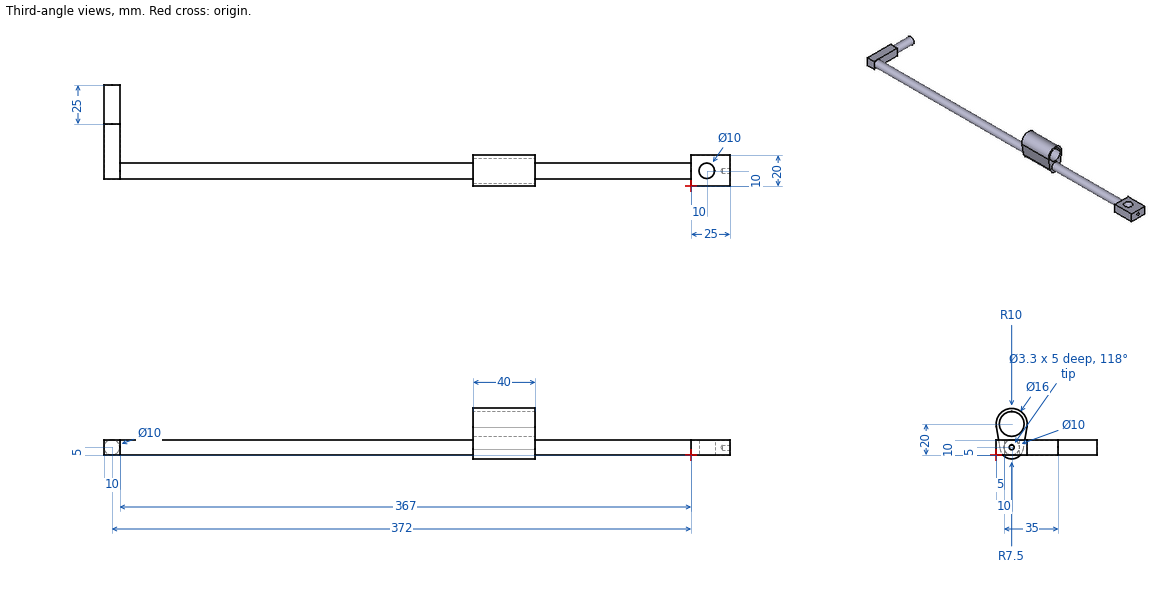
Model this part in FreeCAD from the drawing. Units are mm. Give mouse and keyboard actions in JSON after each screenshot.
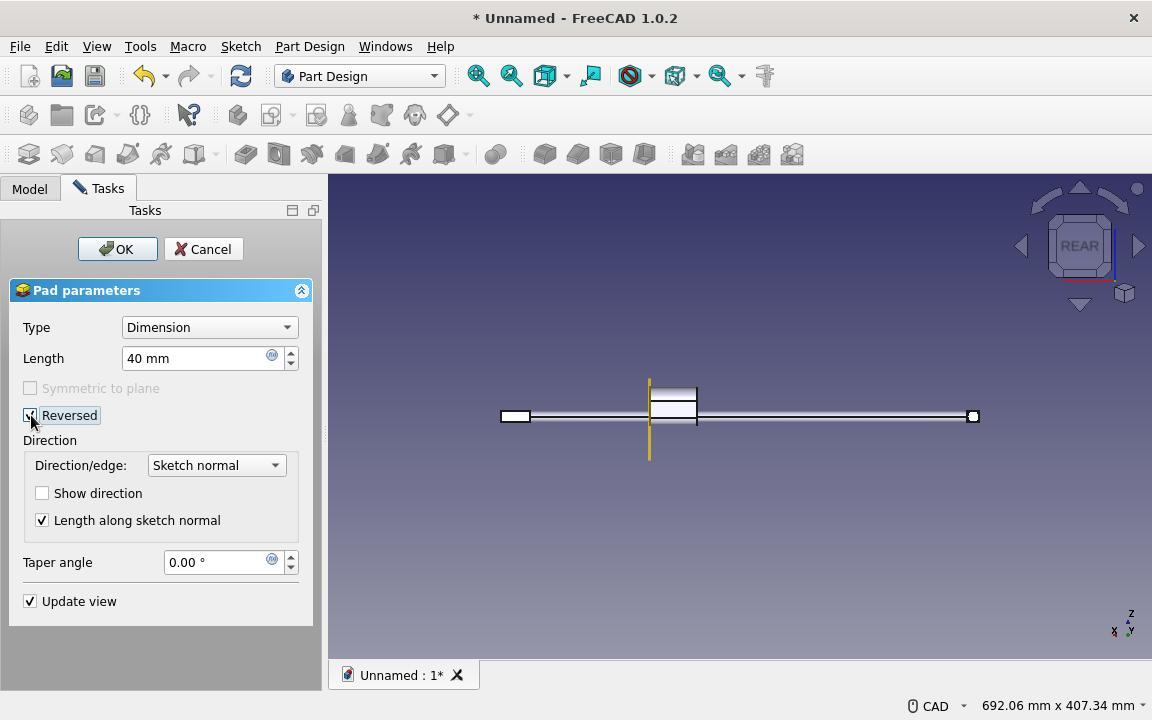
{"action": "left_click", "coordinate": [118, 249]}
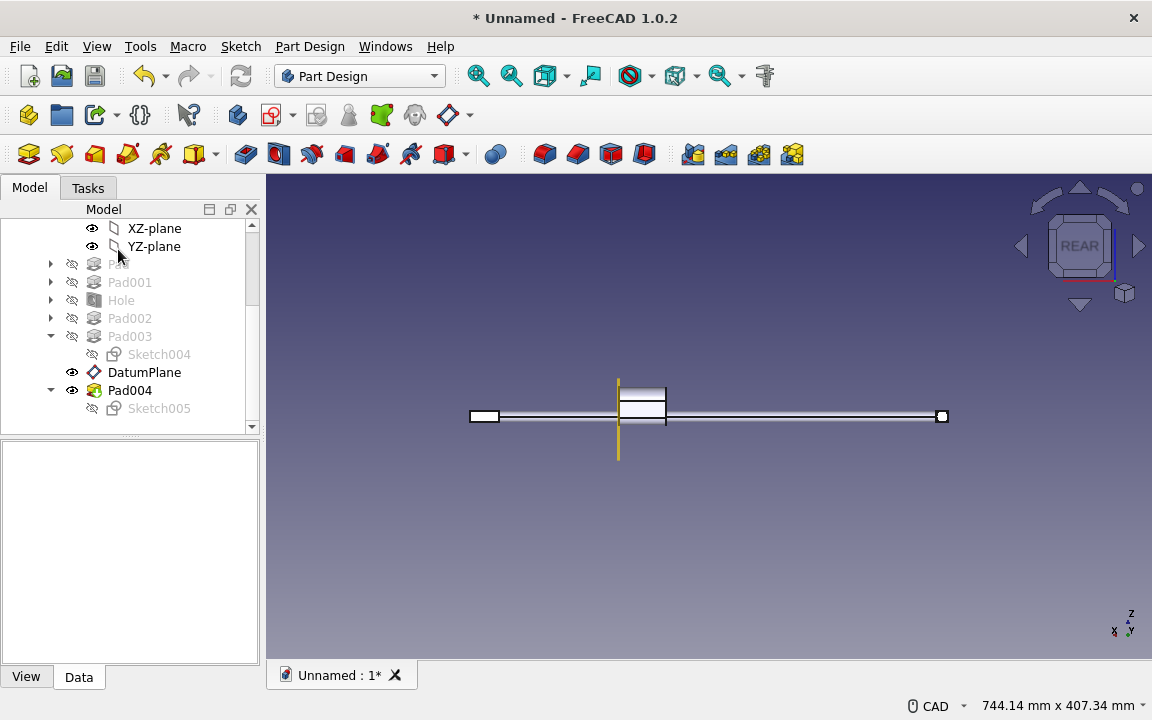
{"action": "left_click", "coordinate": [117, 372]}
{"action": "key", "text": "space"}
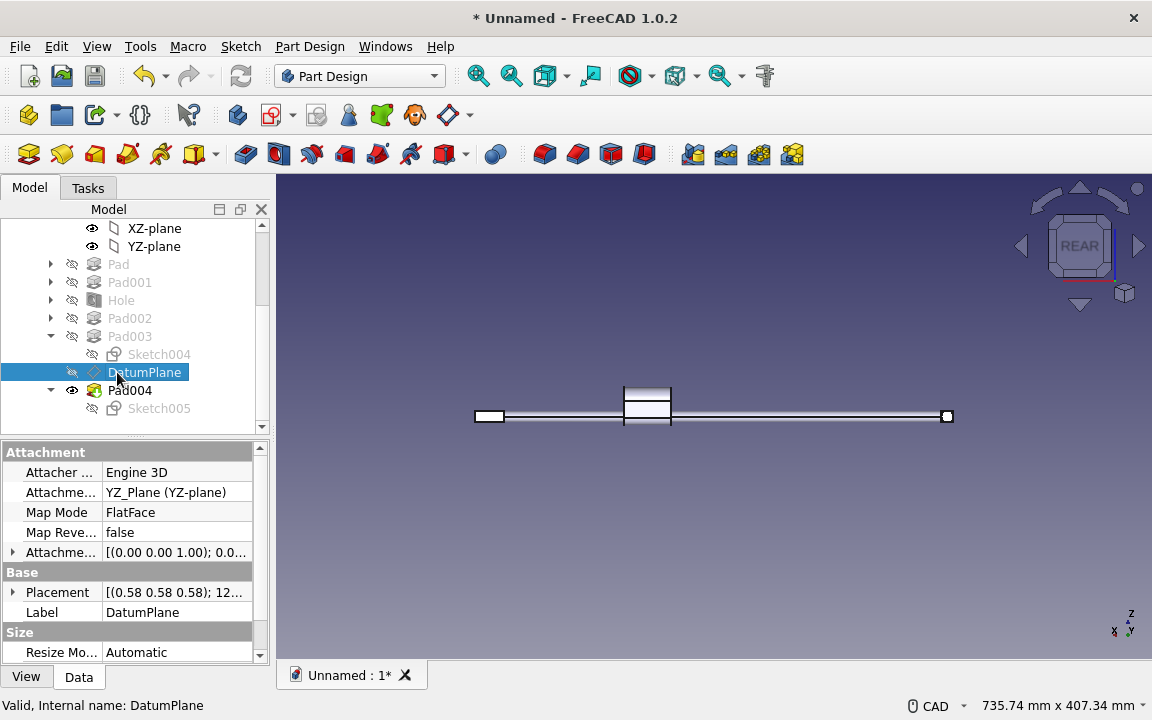
{"action": "key", "text": "0"}